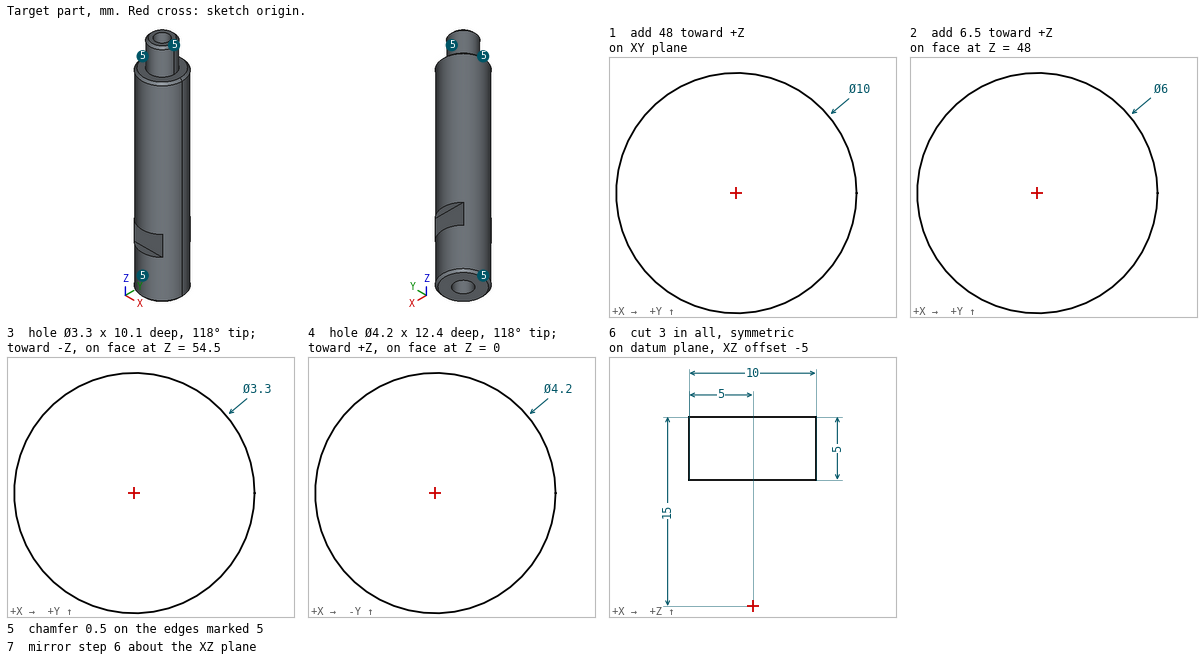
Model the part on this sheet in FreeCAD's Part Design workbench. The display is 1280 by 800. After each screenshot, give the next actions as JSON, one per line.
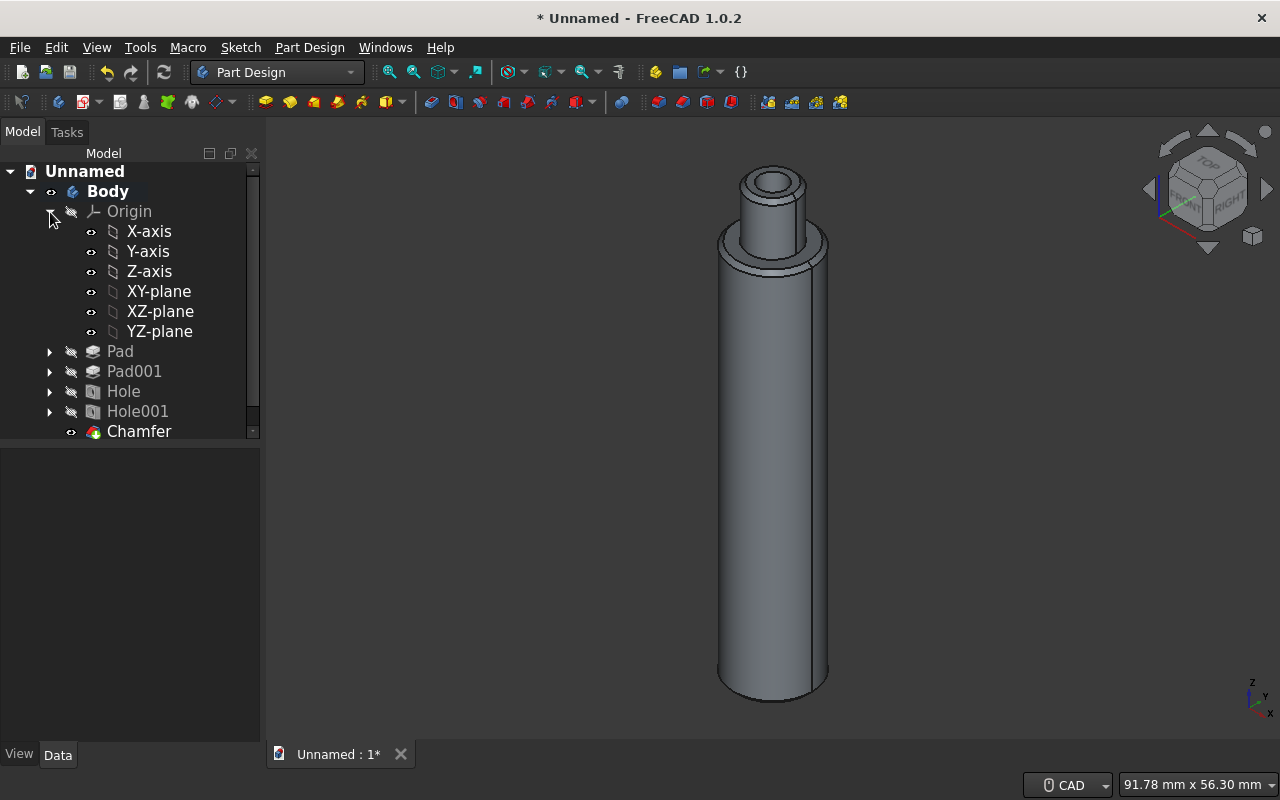
{"action": "left_click", "coordinate": [136, 312]}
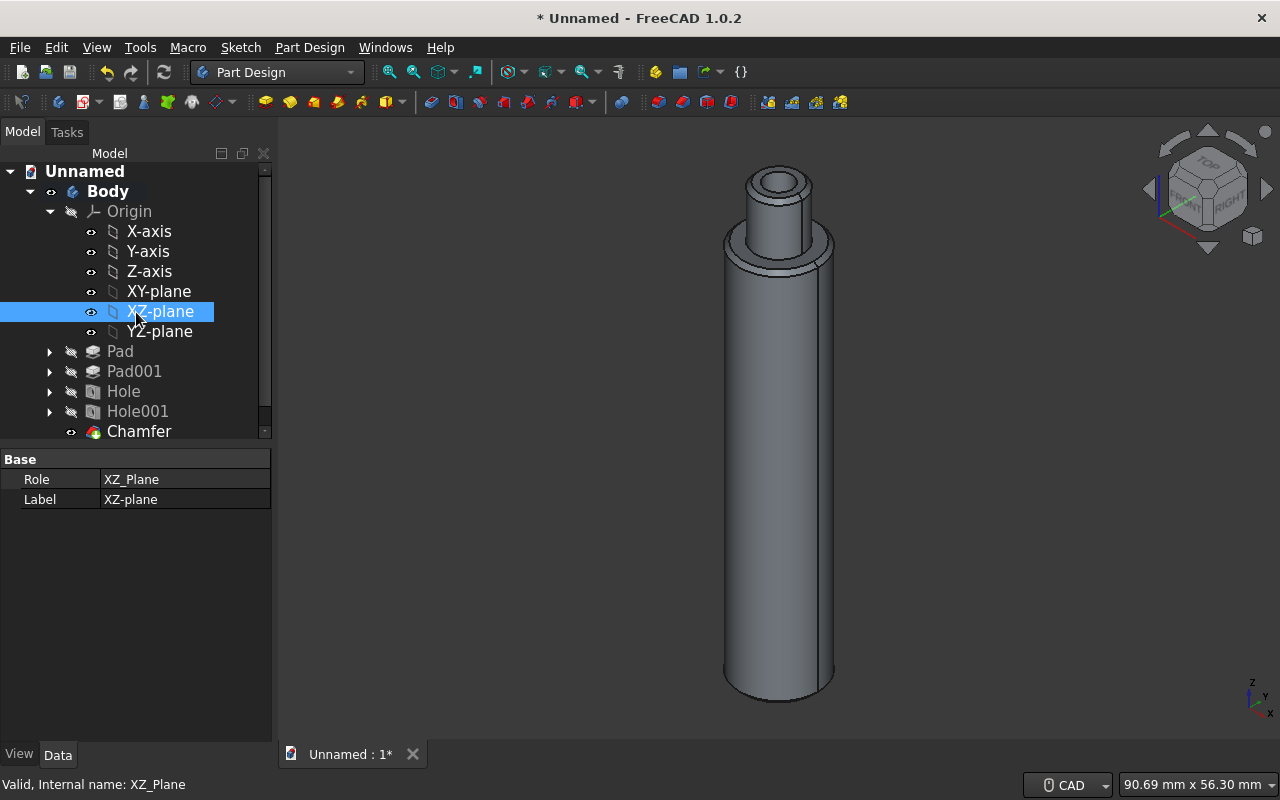
{"action": "left_click", "coordinate": [216, 102]}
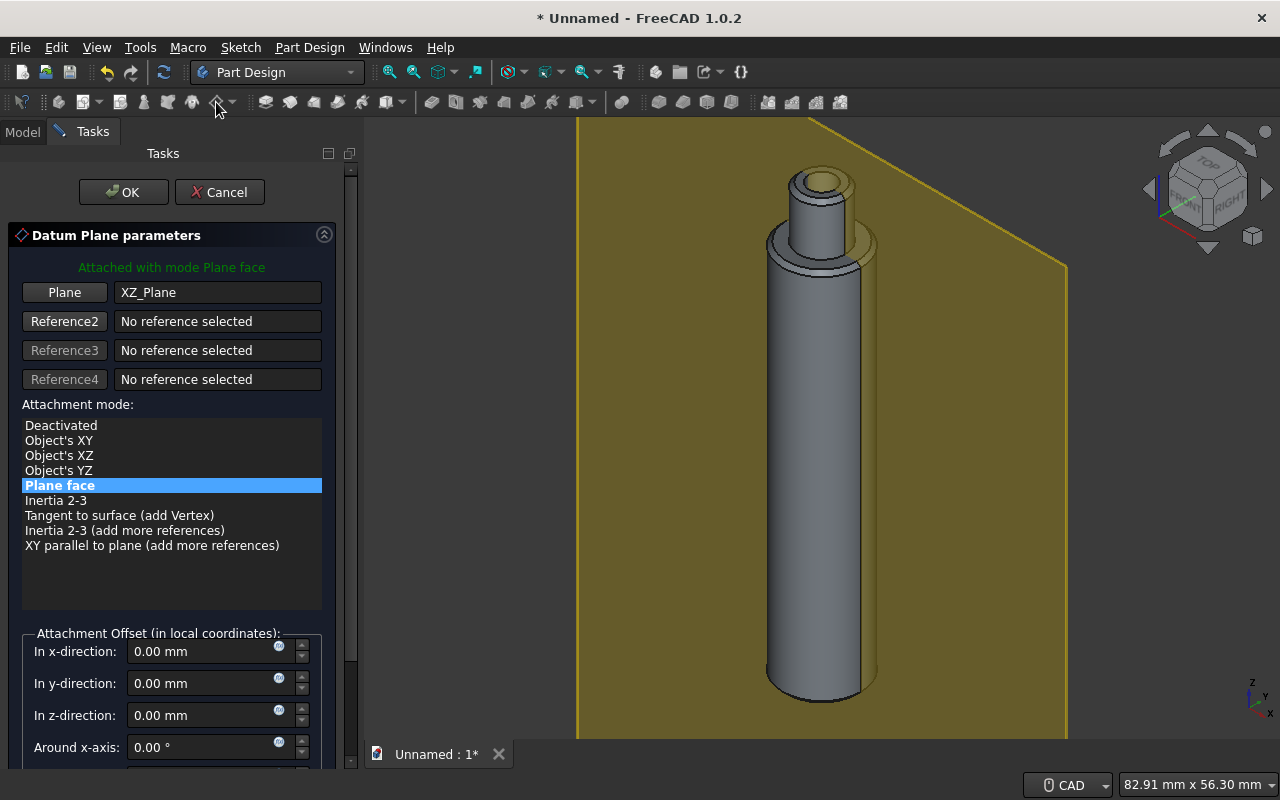
{"action": "triple_click", "coordinate": [210, 715]}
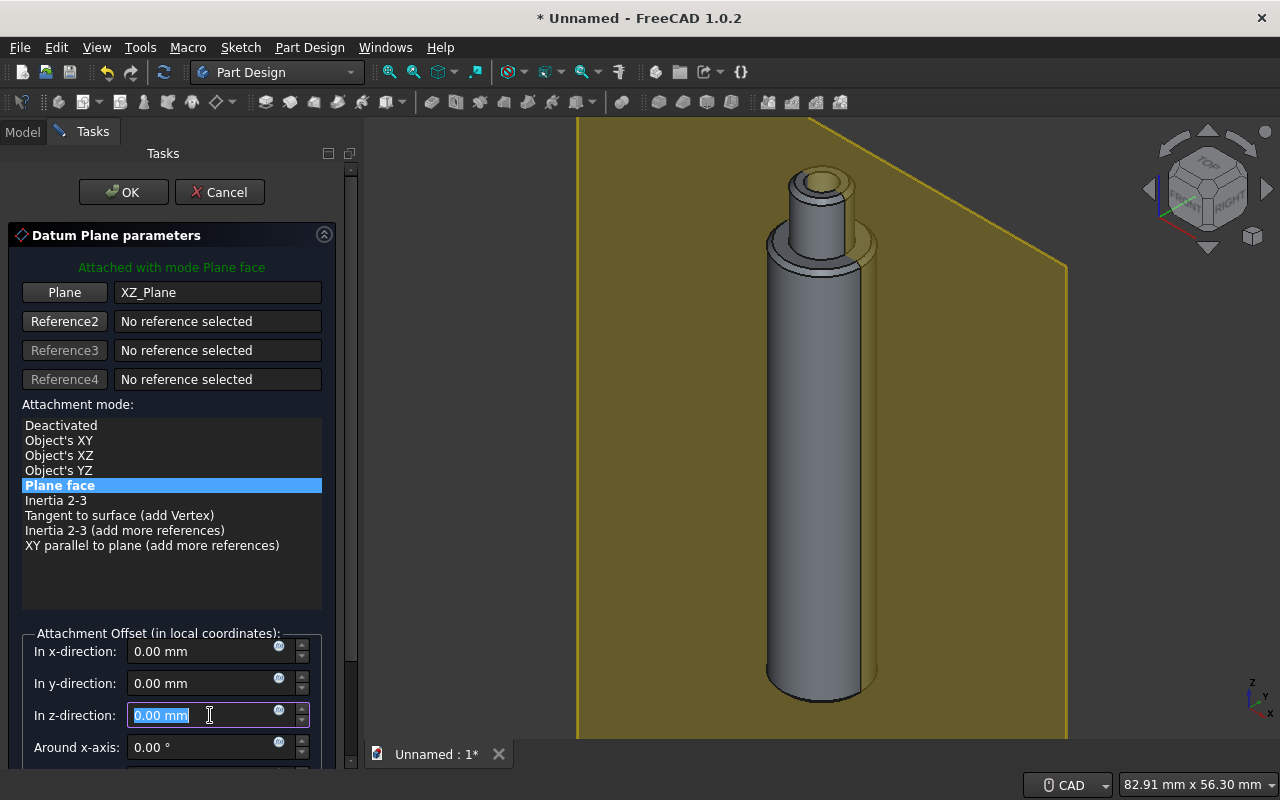
{"action": "type", "text": "-5"}
{"action": "key", "text": "Tab"}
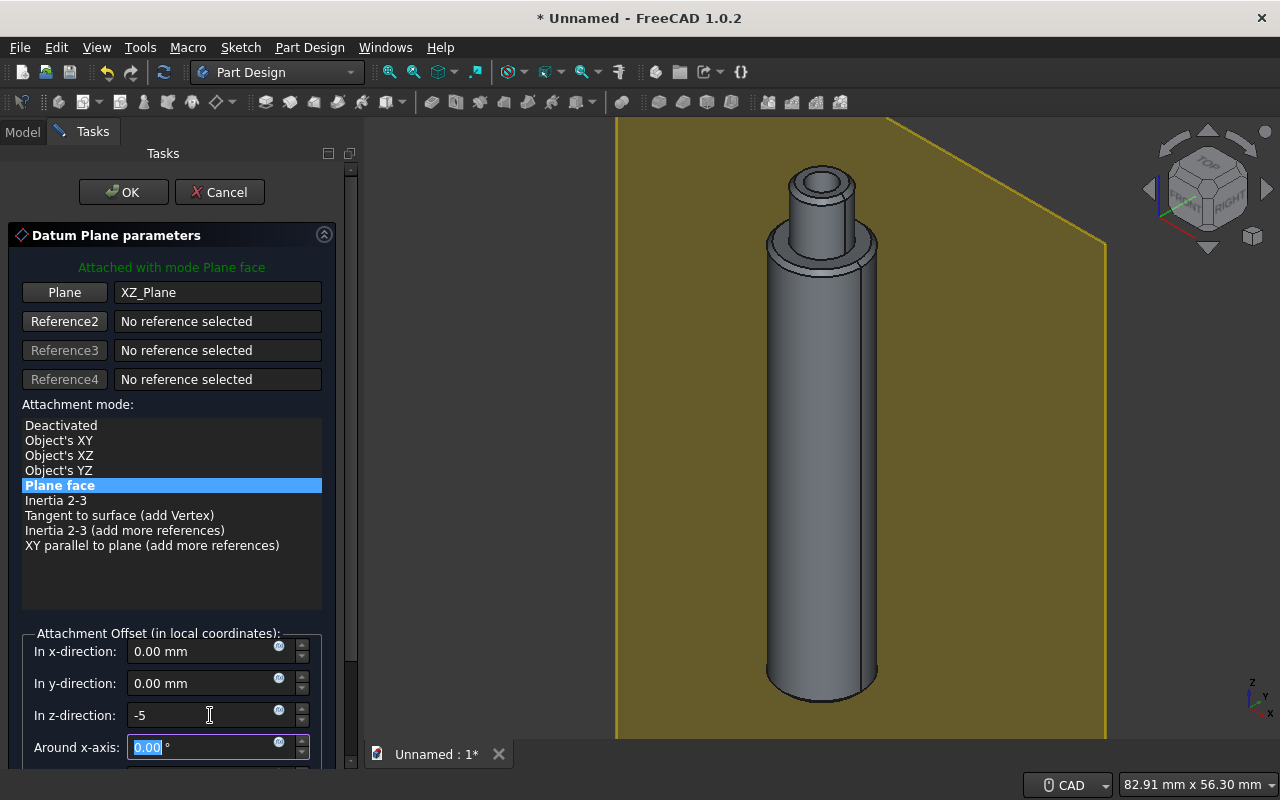
{"action": "left_click", "coordinate": [124, 192]}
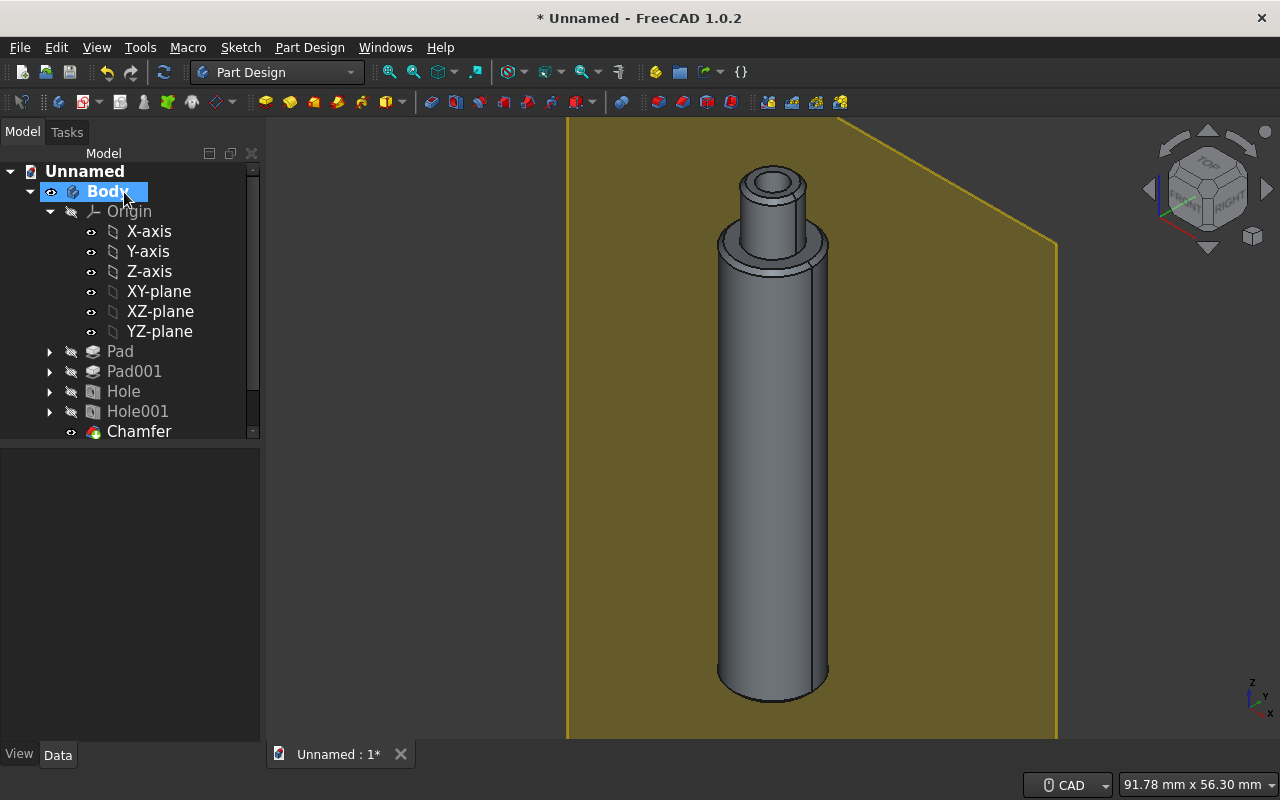
{"action": "scroll", "coordinate": [100, 307], "scroll_direction": "down", "scroll_amount": 3}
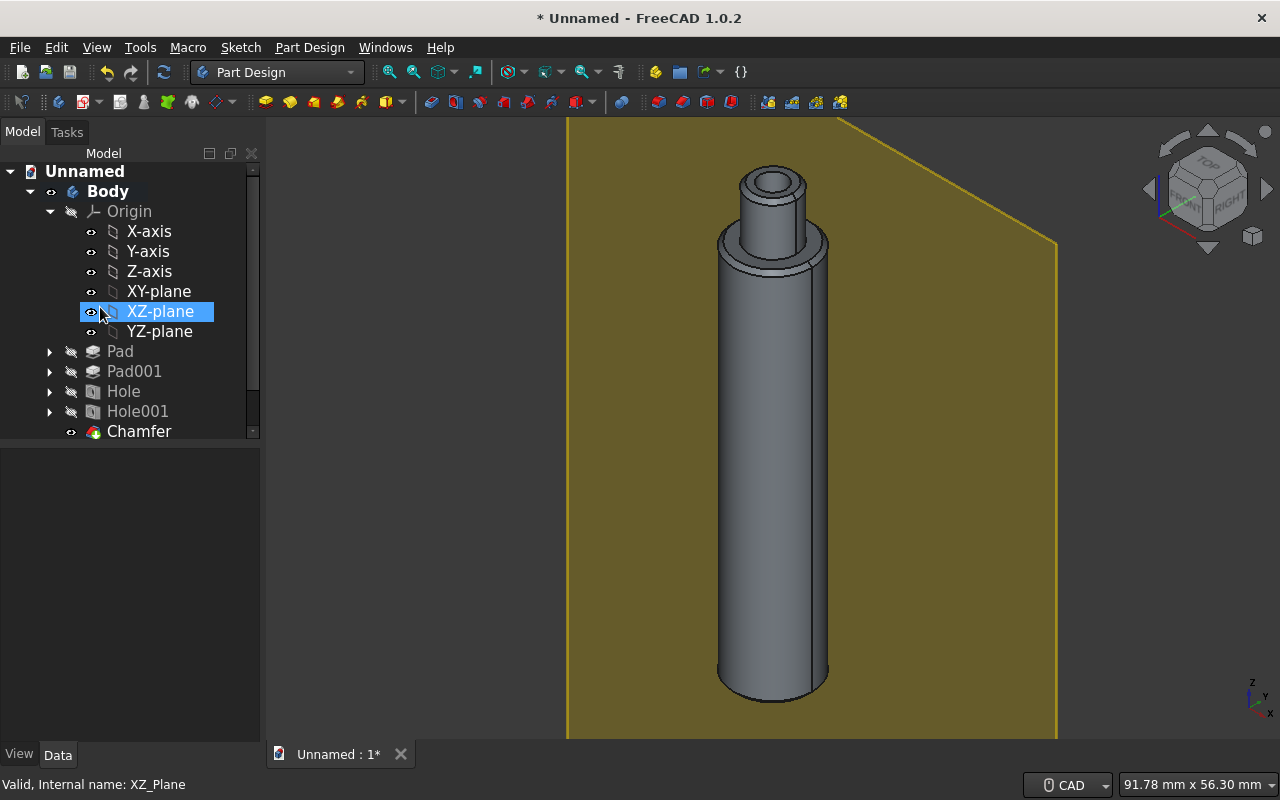
{"action": "left_click", "coordinate": [116, 412]}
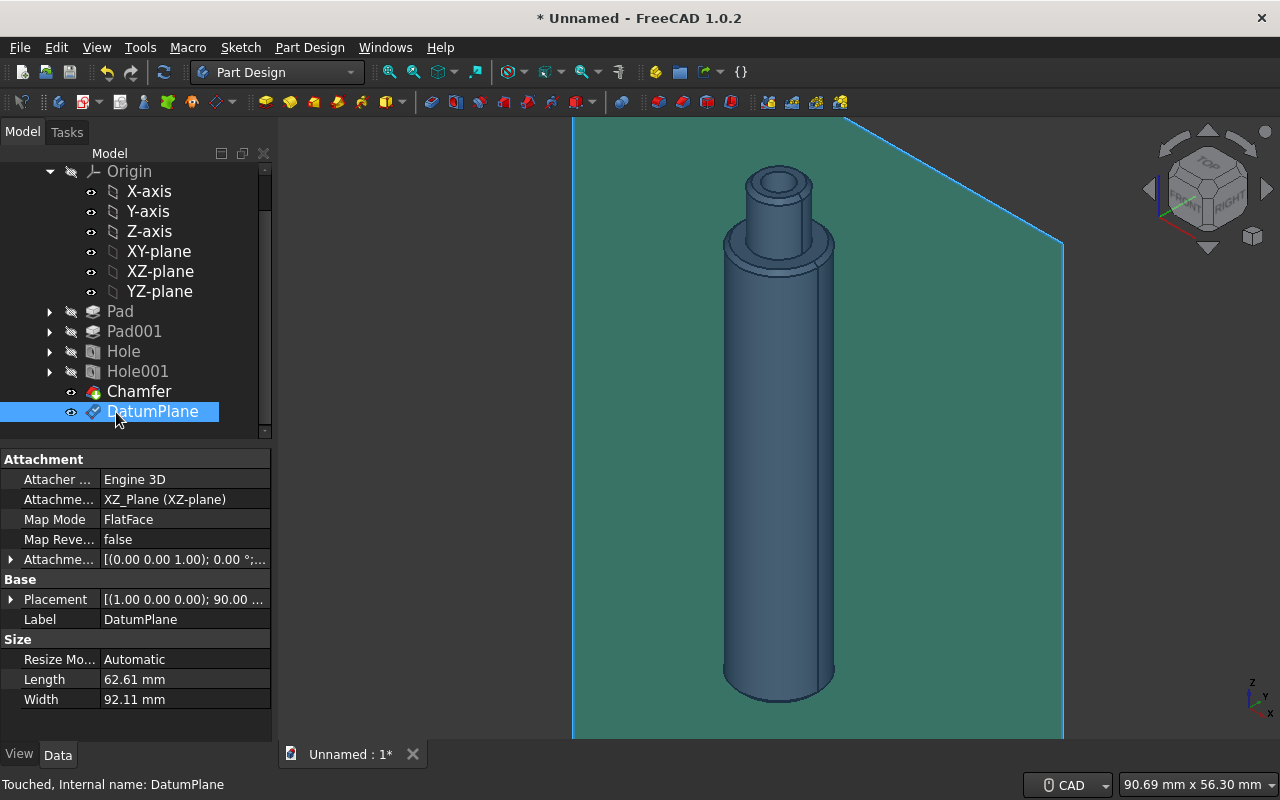
{"action": "left_click", "coordinate": [84, 102]}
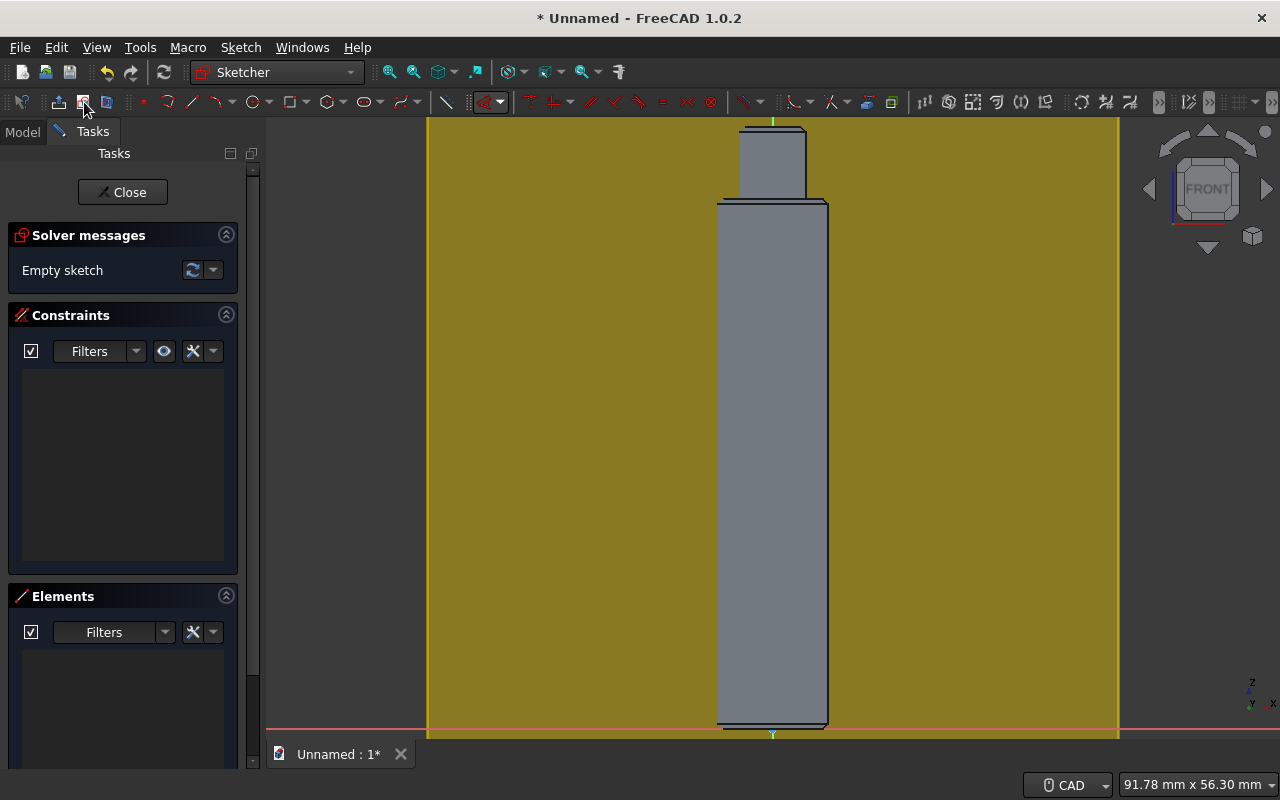
{"action": "key", "text": "q s"}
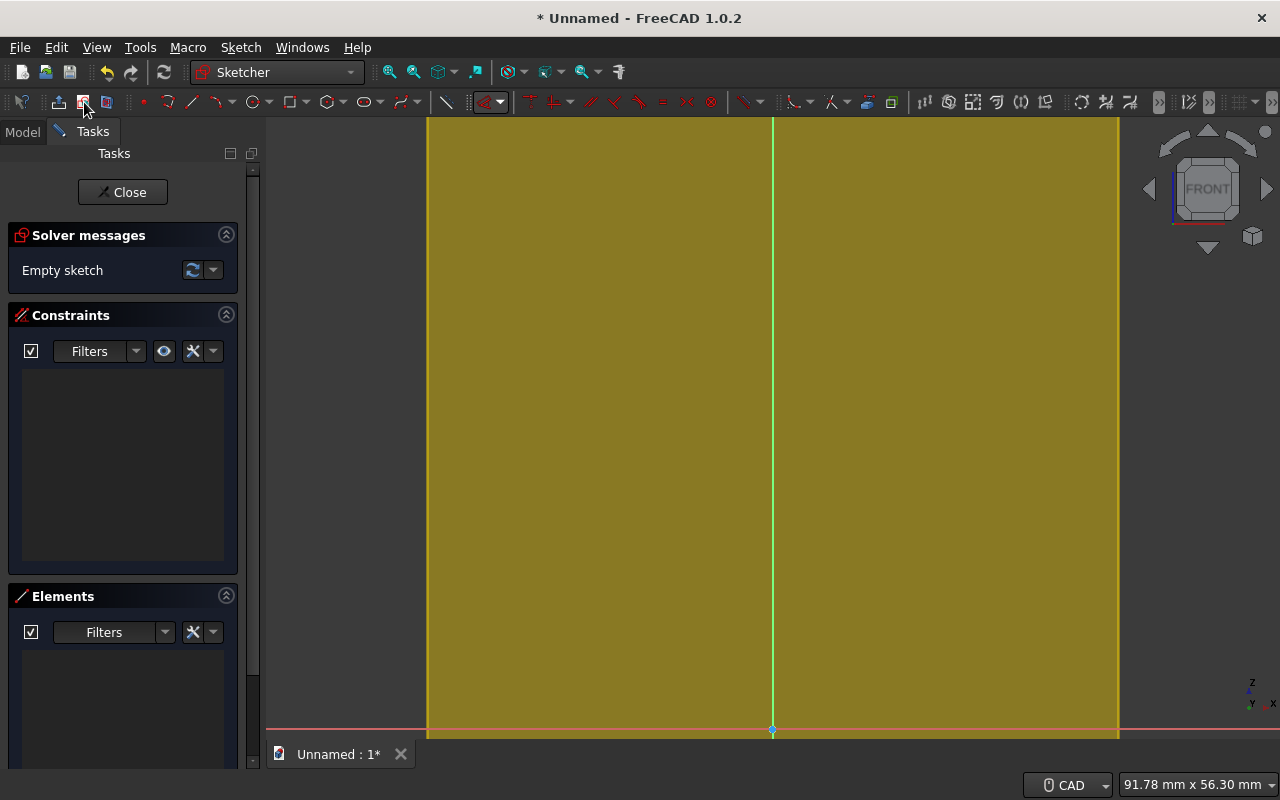
{"action": "scroll", "coordinate": [704, 428], "scroll_direction": "down", "scroll_amount": 5}